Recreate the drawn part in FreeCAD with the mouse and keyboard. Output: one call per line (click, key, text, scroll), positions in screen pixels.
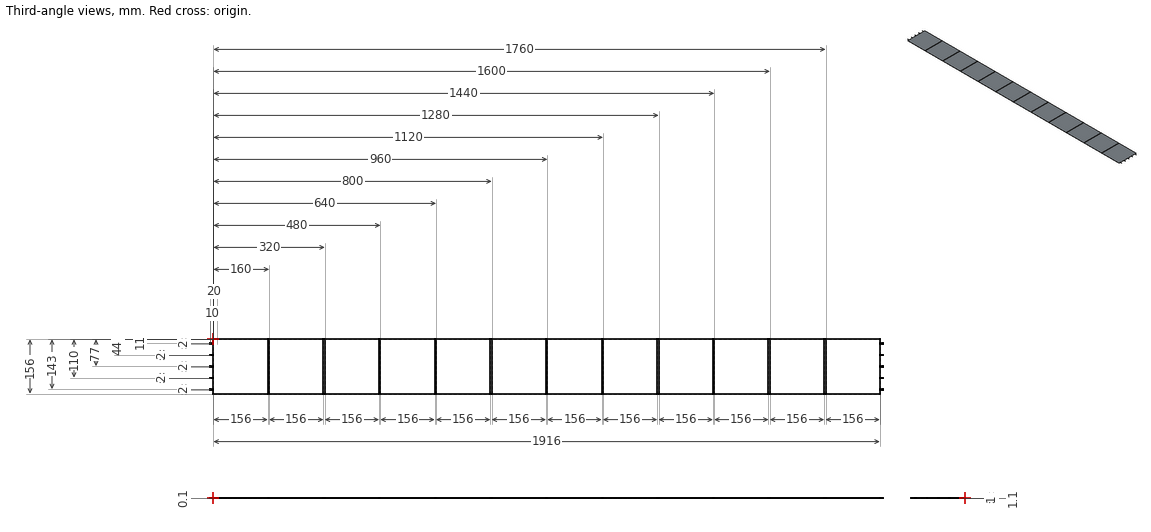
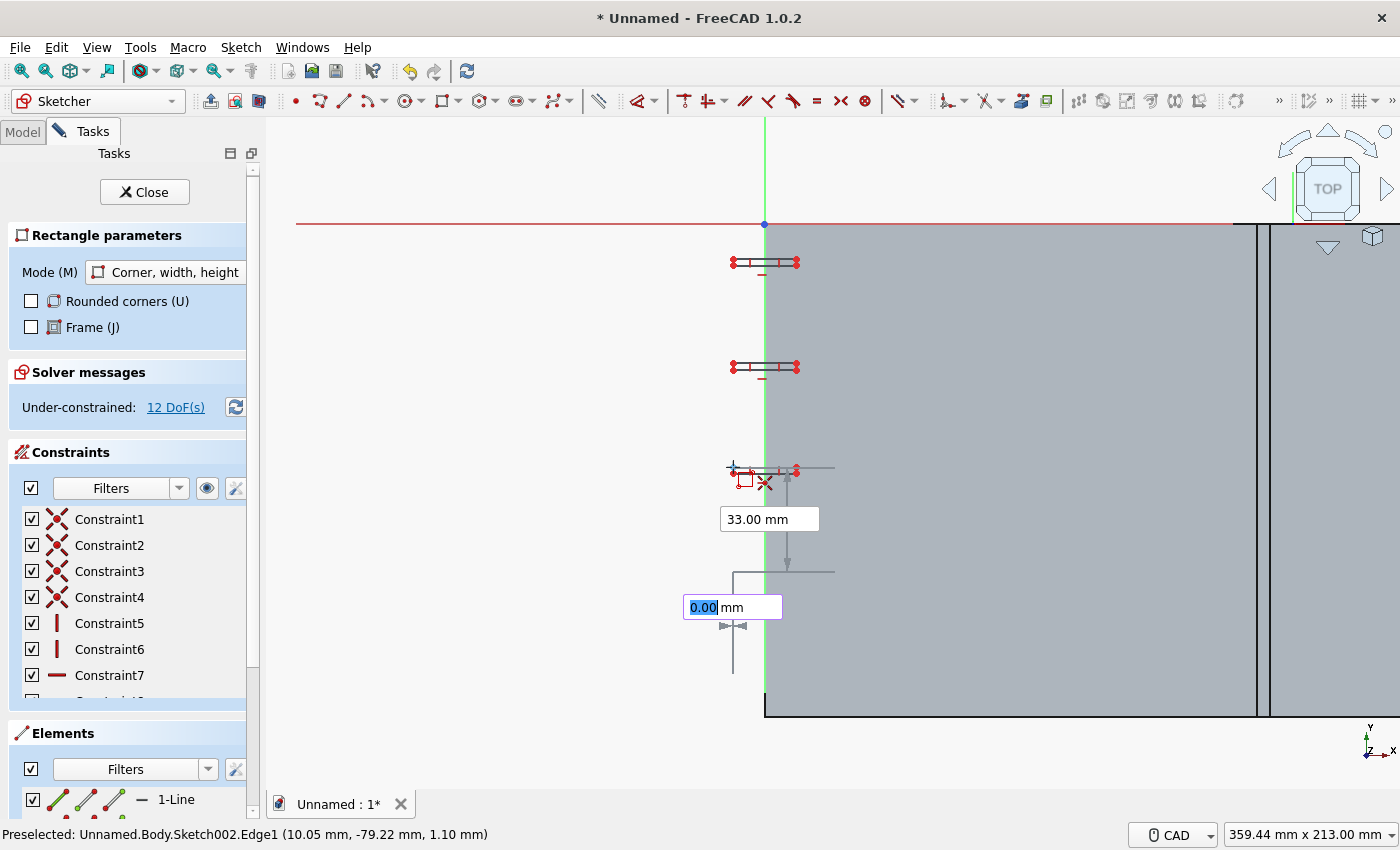
click(796, 578)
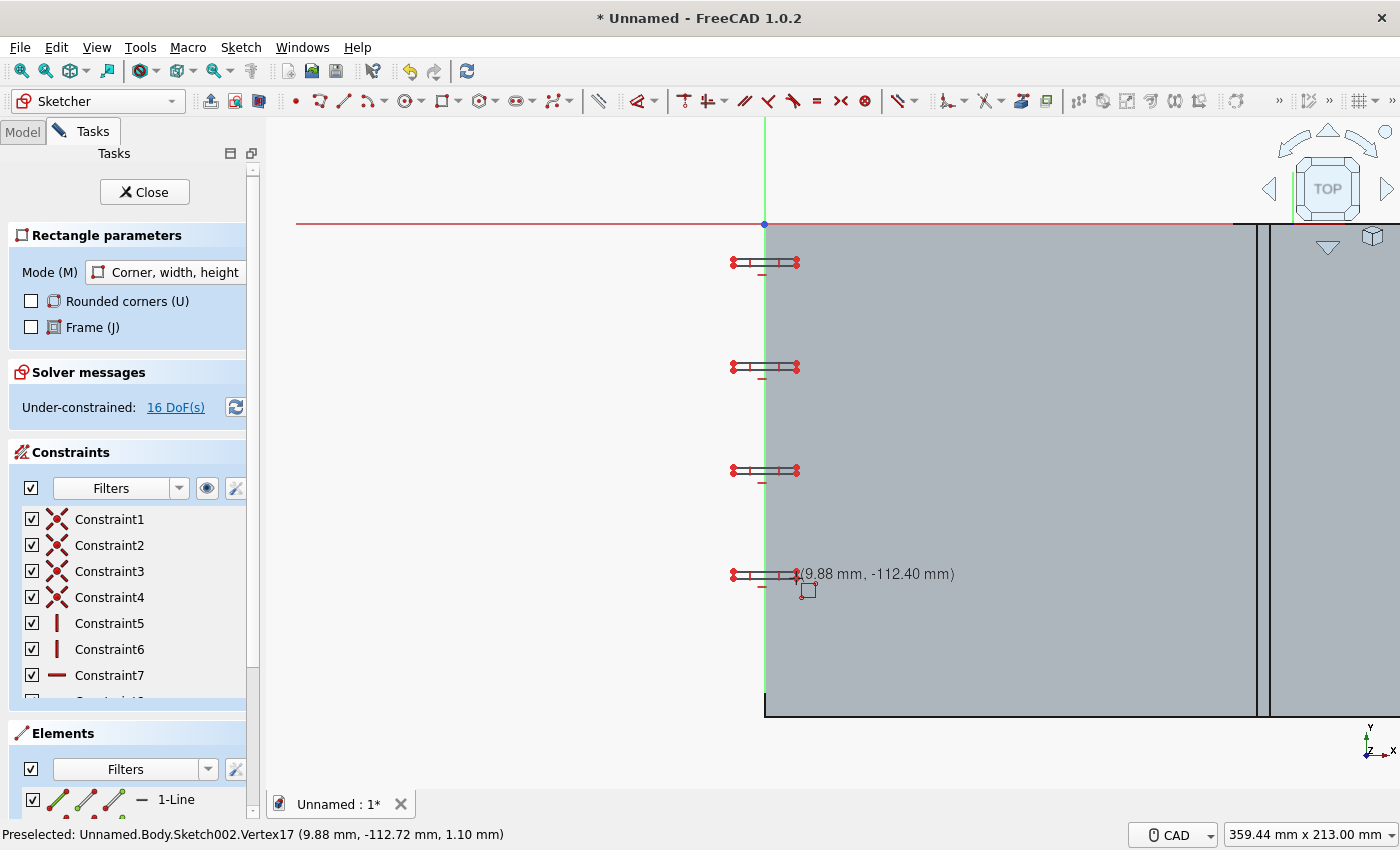
scroll(733, 676, up, 5)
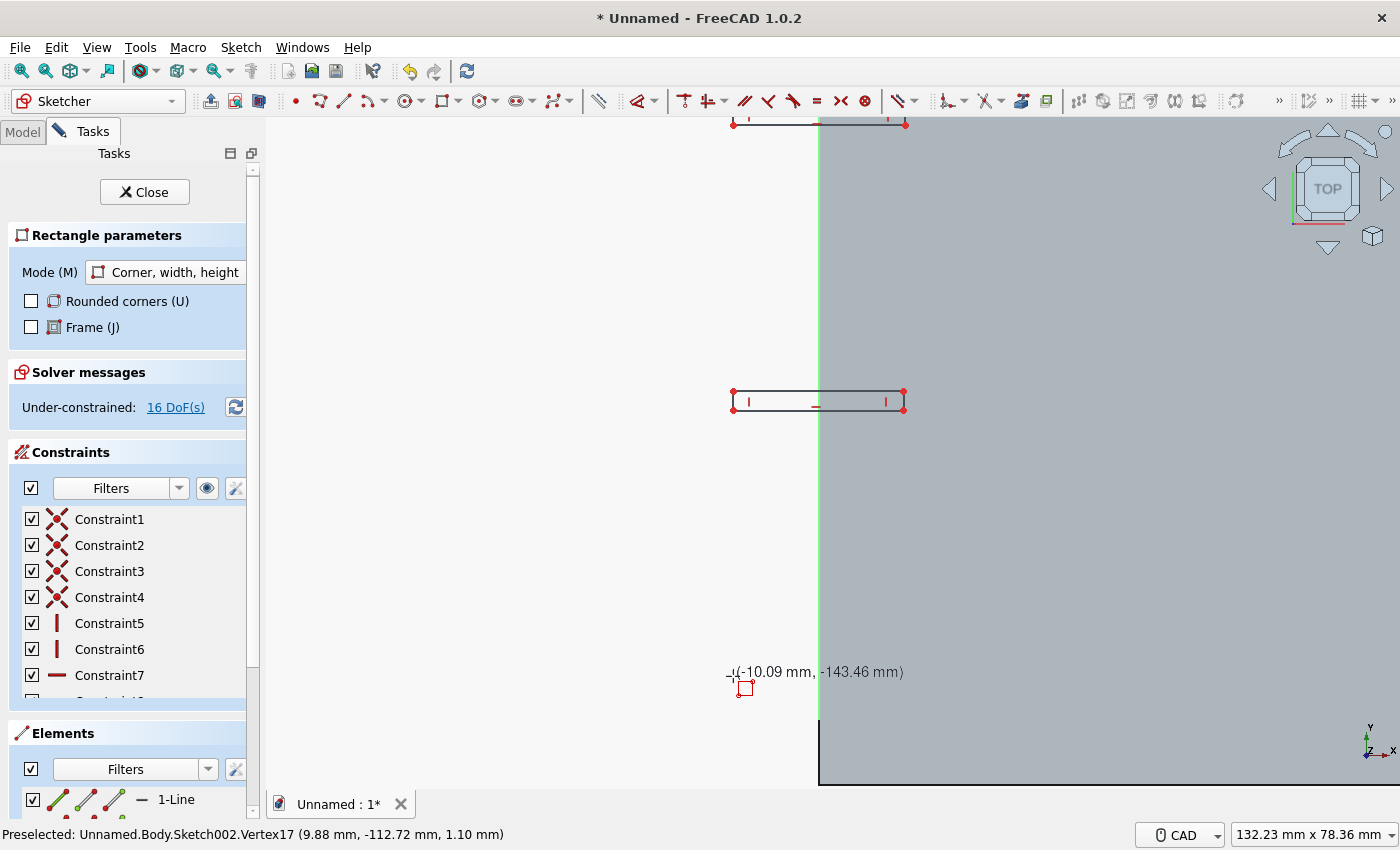
click(733, 673)
click(905, 690)
key(Escape)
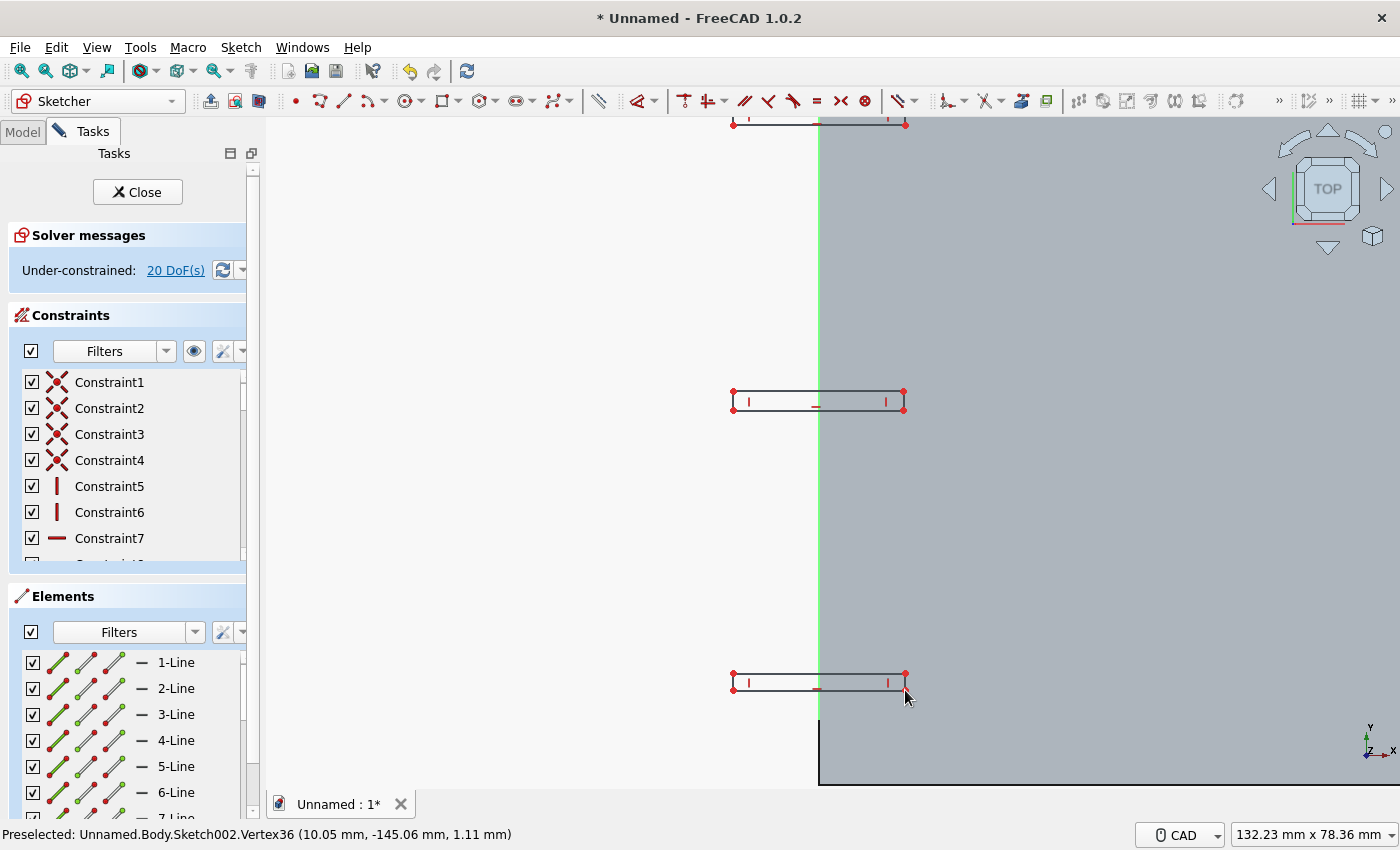
click(638, 102)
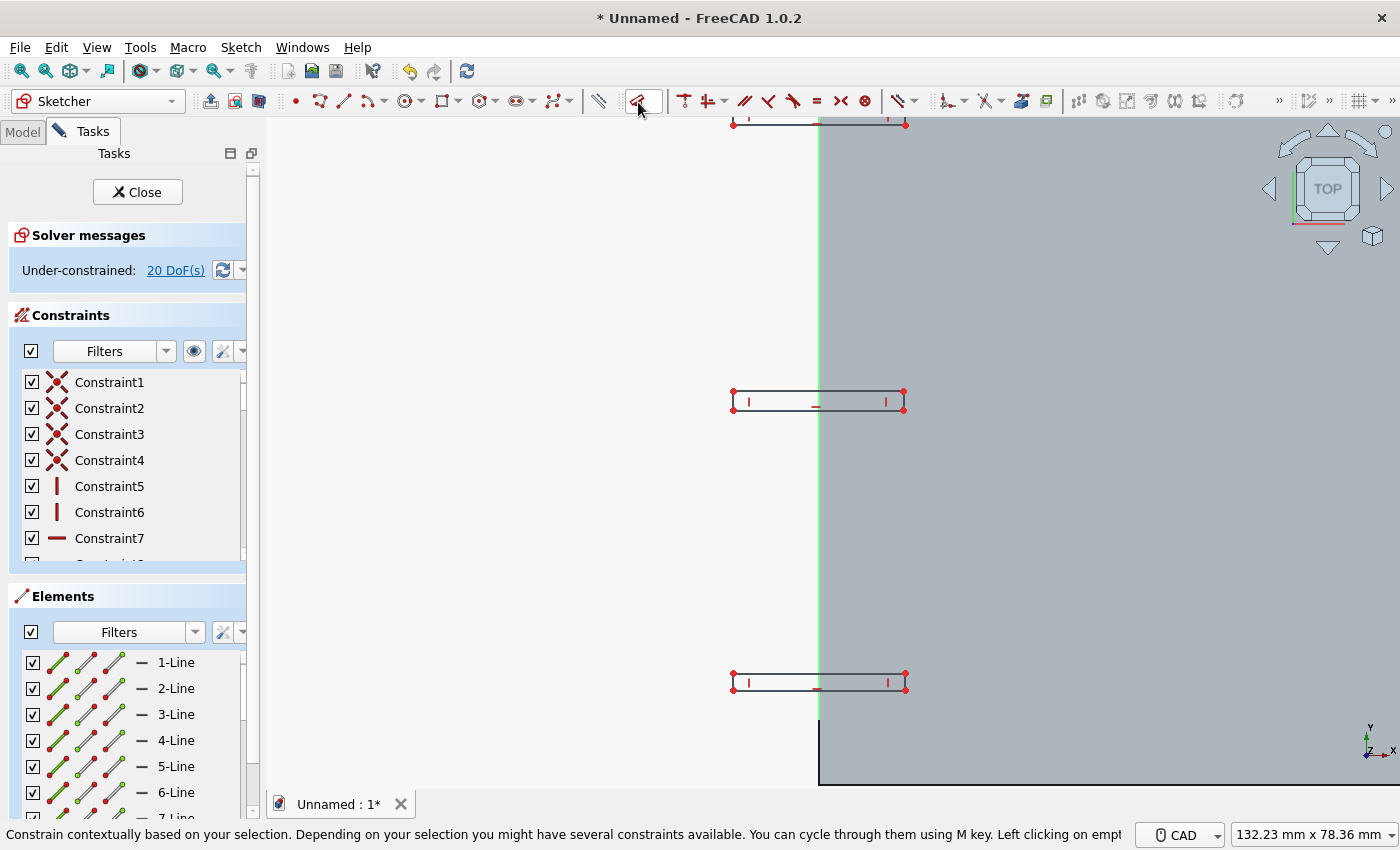
scroll(733, 677, down, 5)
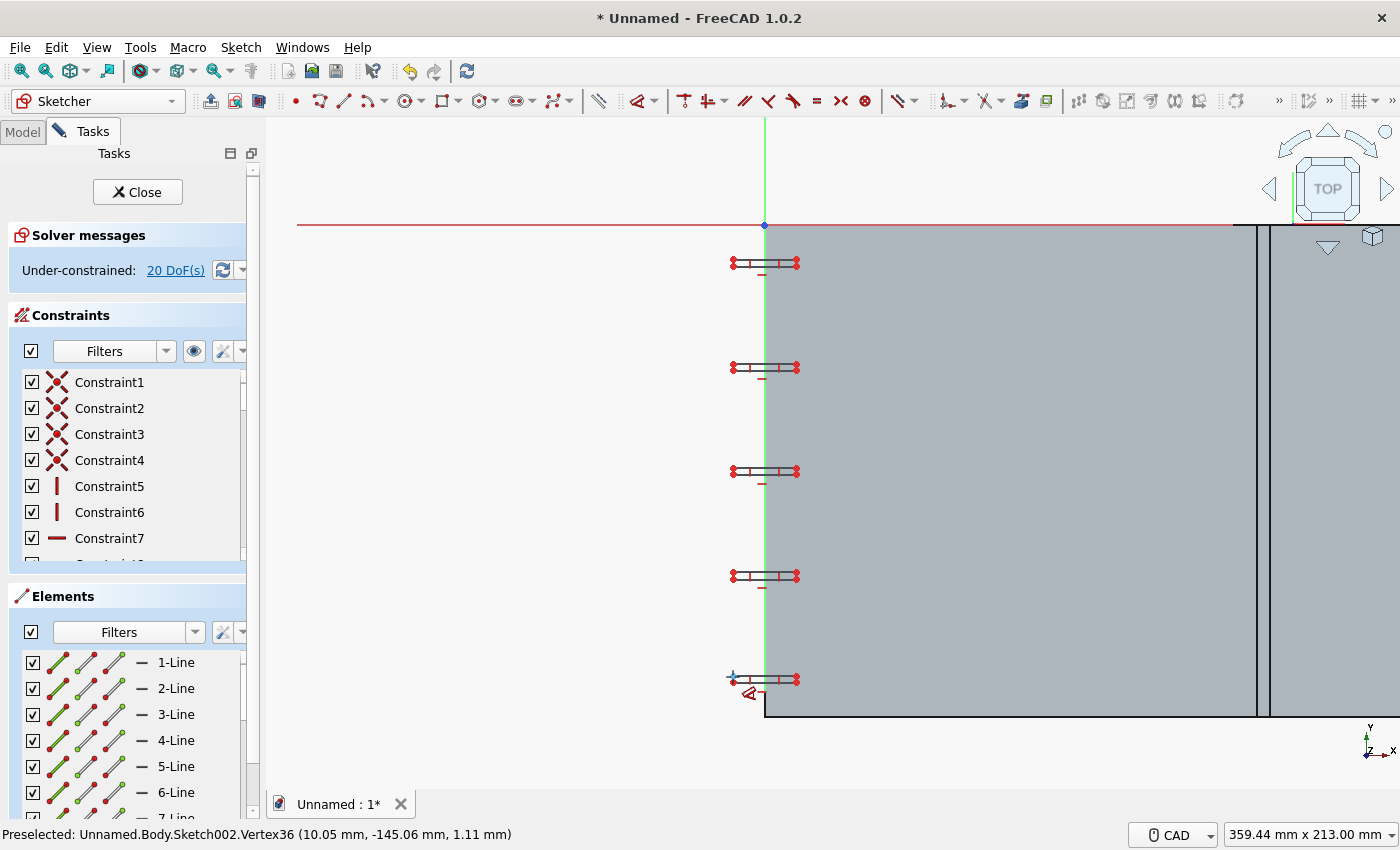
scroll(733, 263, up, 10)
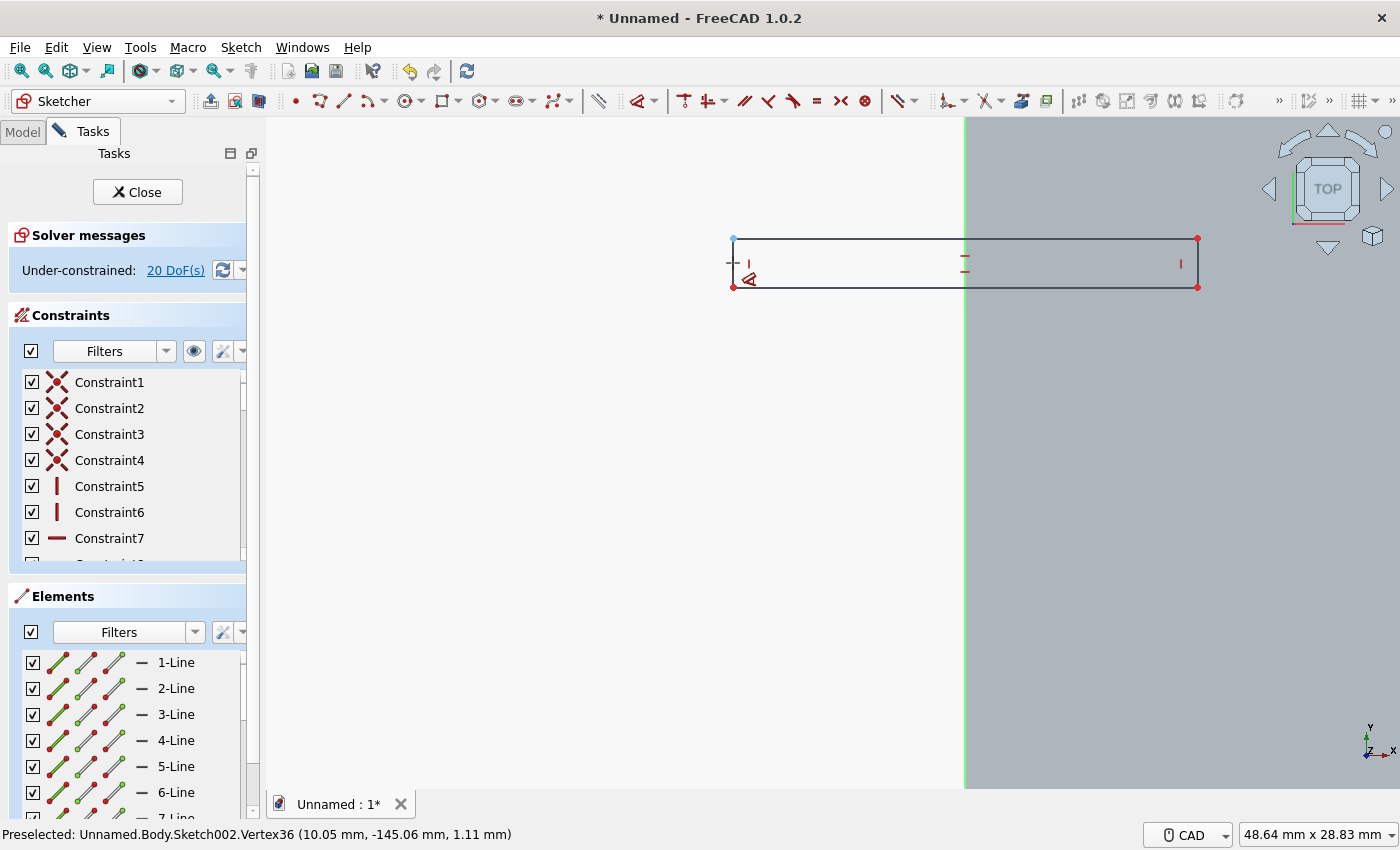
click(733, 263)
click(699, 263)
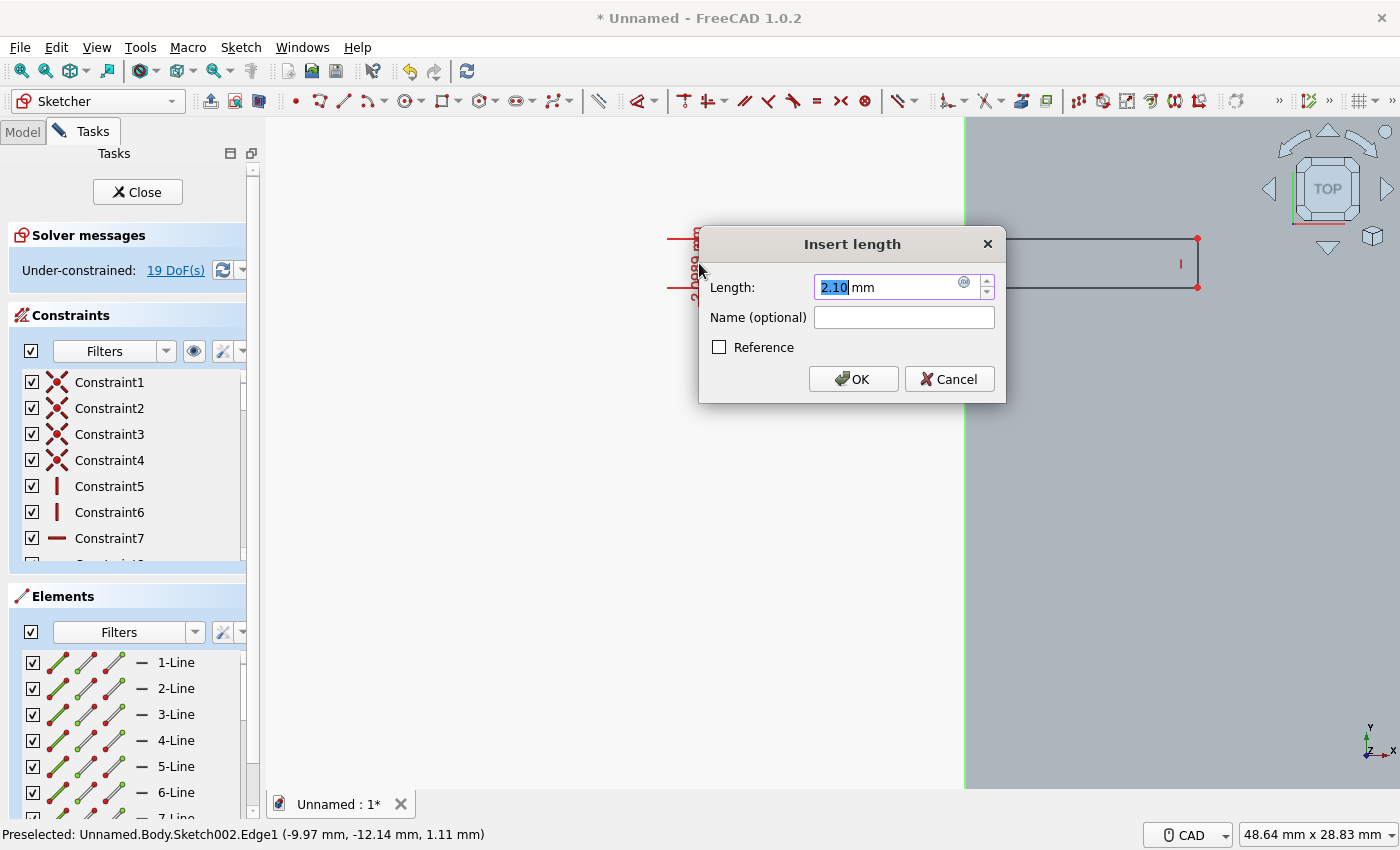
text(2)
key(Return)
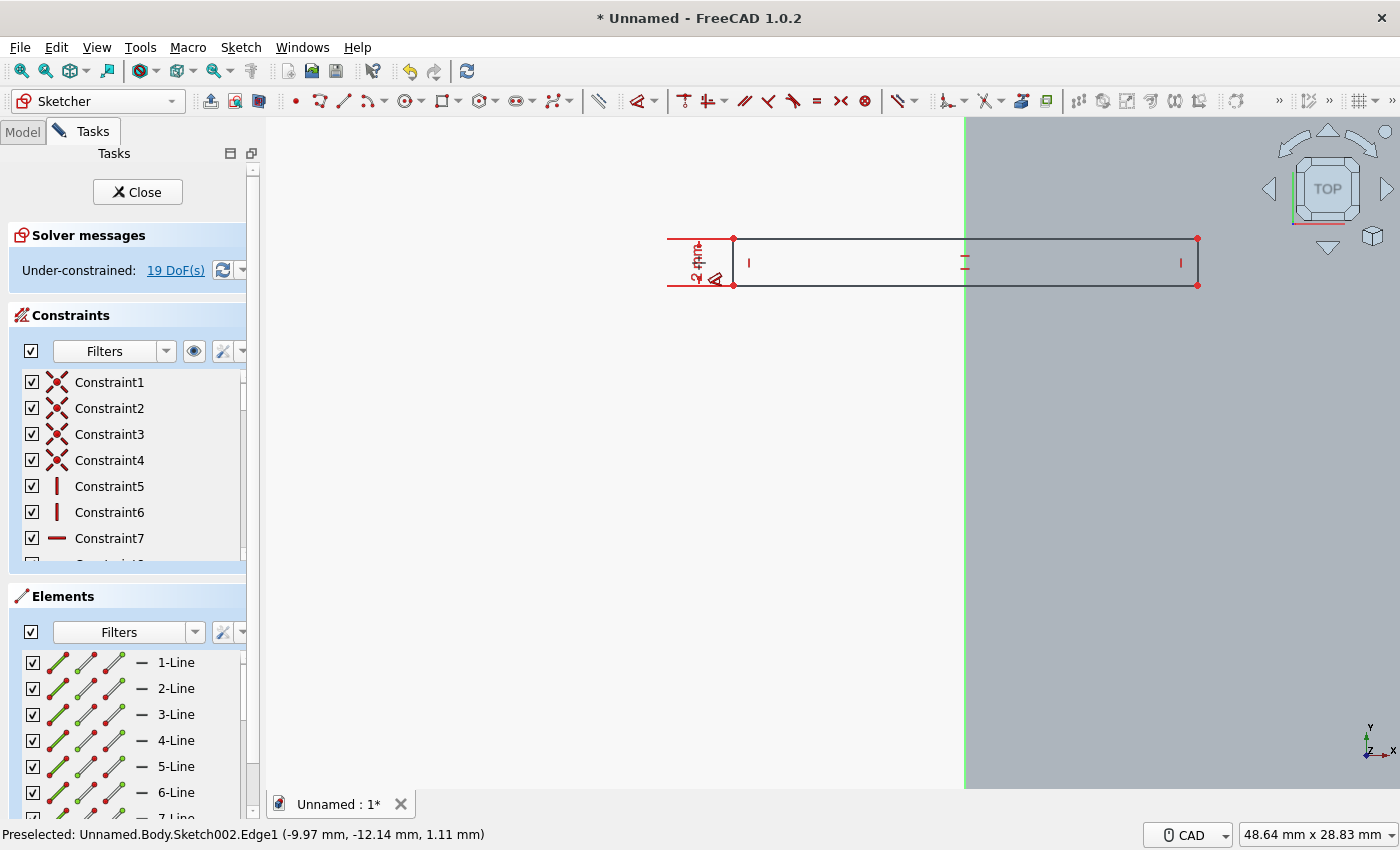
scroll(733, 262, down, 10)